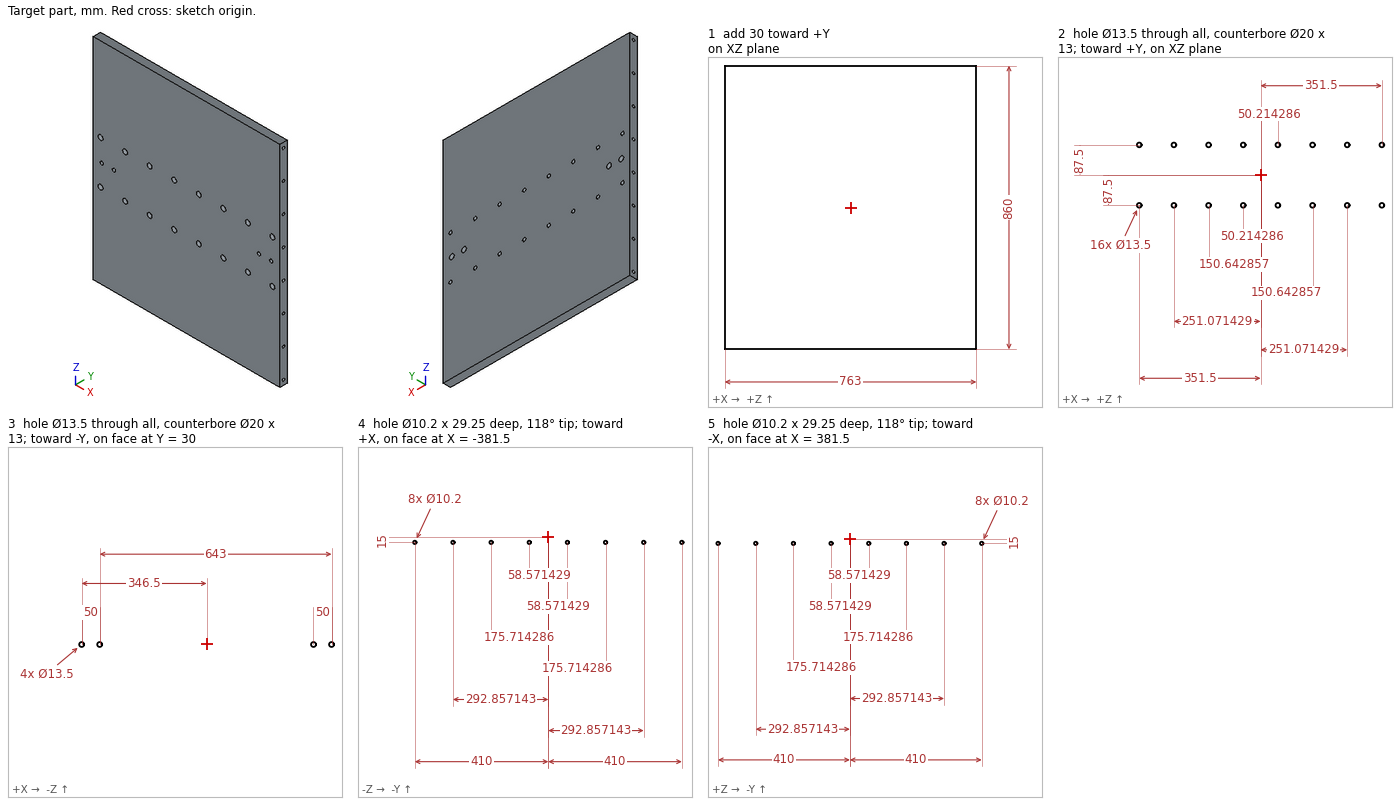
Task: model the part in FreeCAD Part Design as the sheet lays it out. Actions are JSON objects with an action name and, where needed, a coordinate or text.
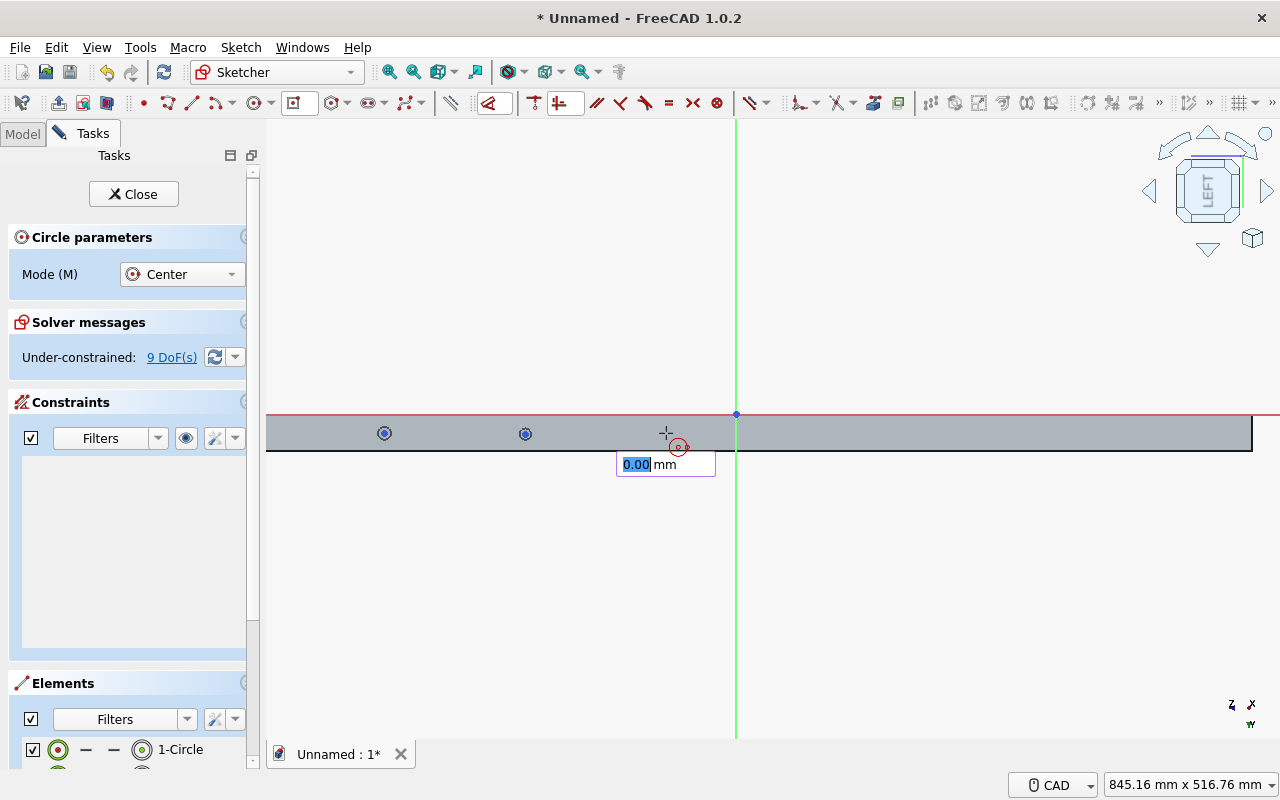
{"action": "scroll", "coordinate": [670, 437], "scroll_direction": "up", "scroll_amount": 5}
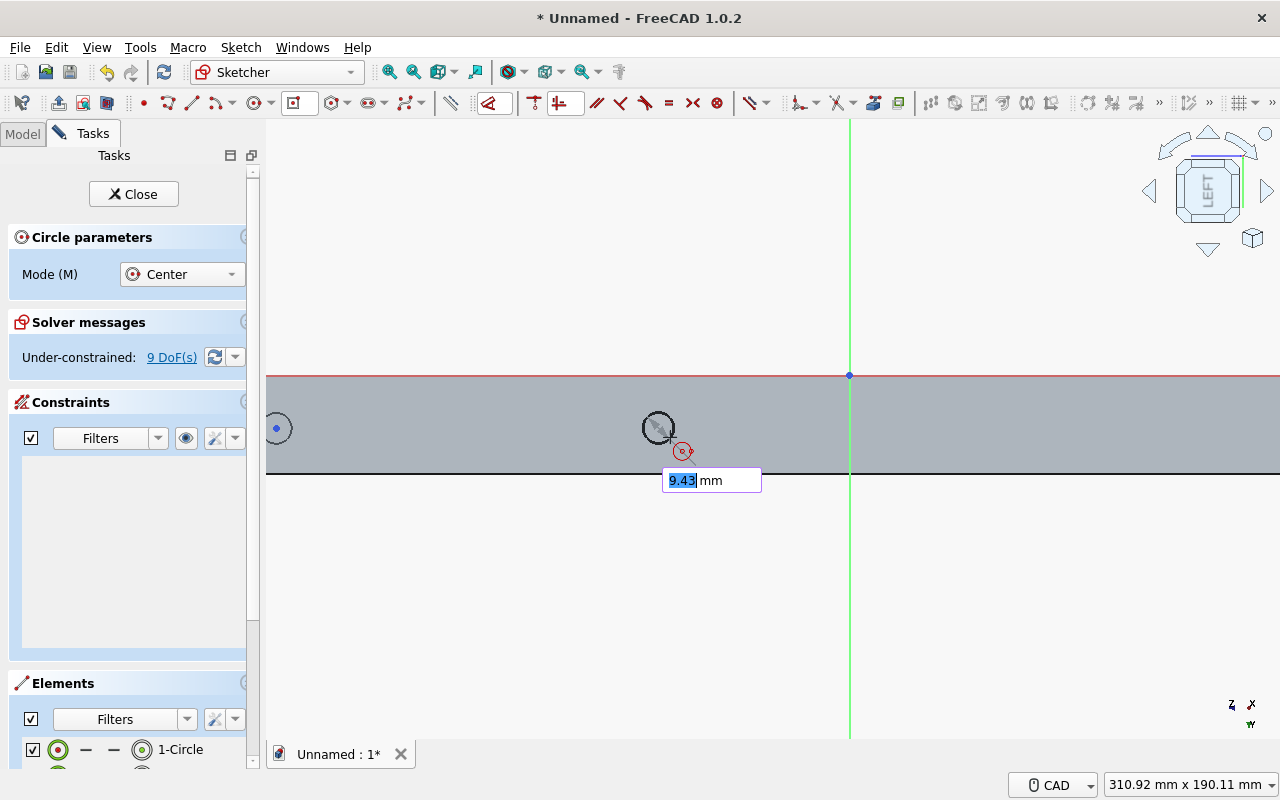
{"action": "left_click", "coordinate": [670, 436]}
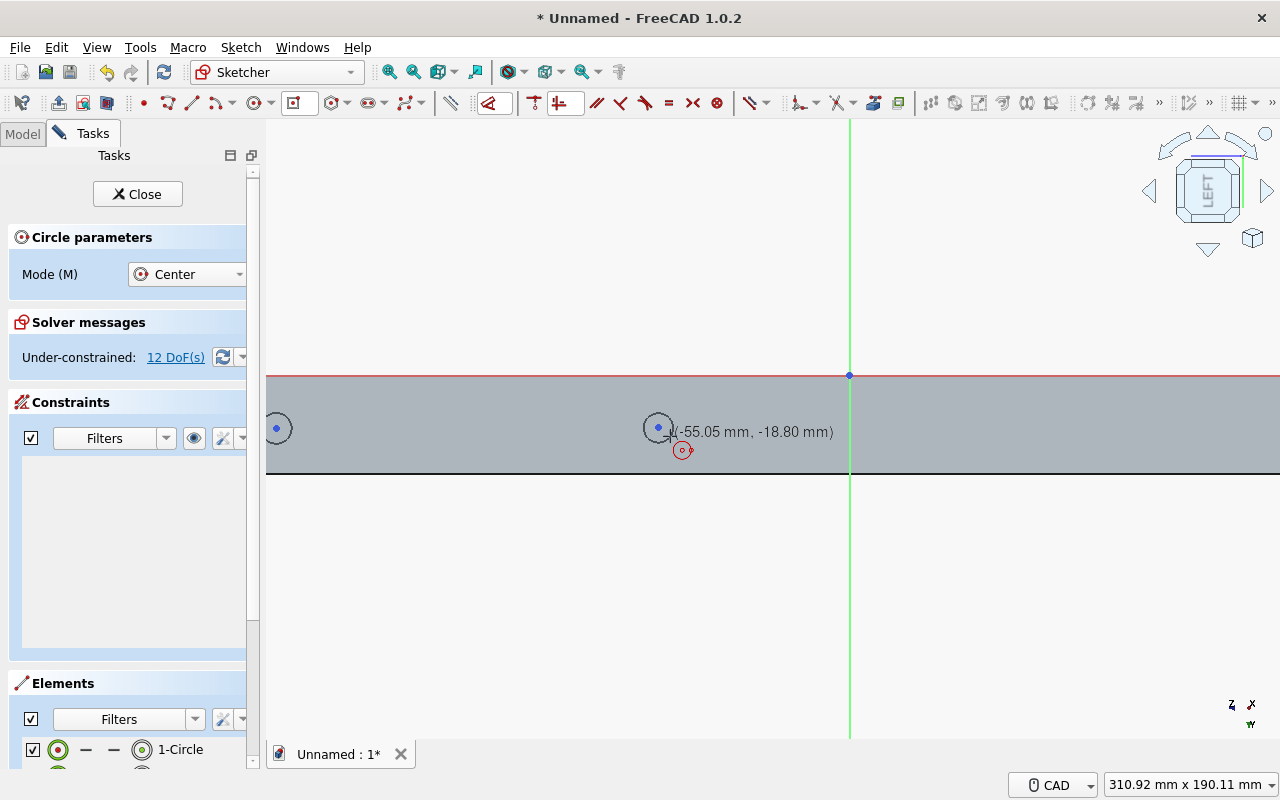
{"action": "scroll", "coordinate": [1041, 425], "scroll_direction": "up", "scroll_amount": 2}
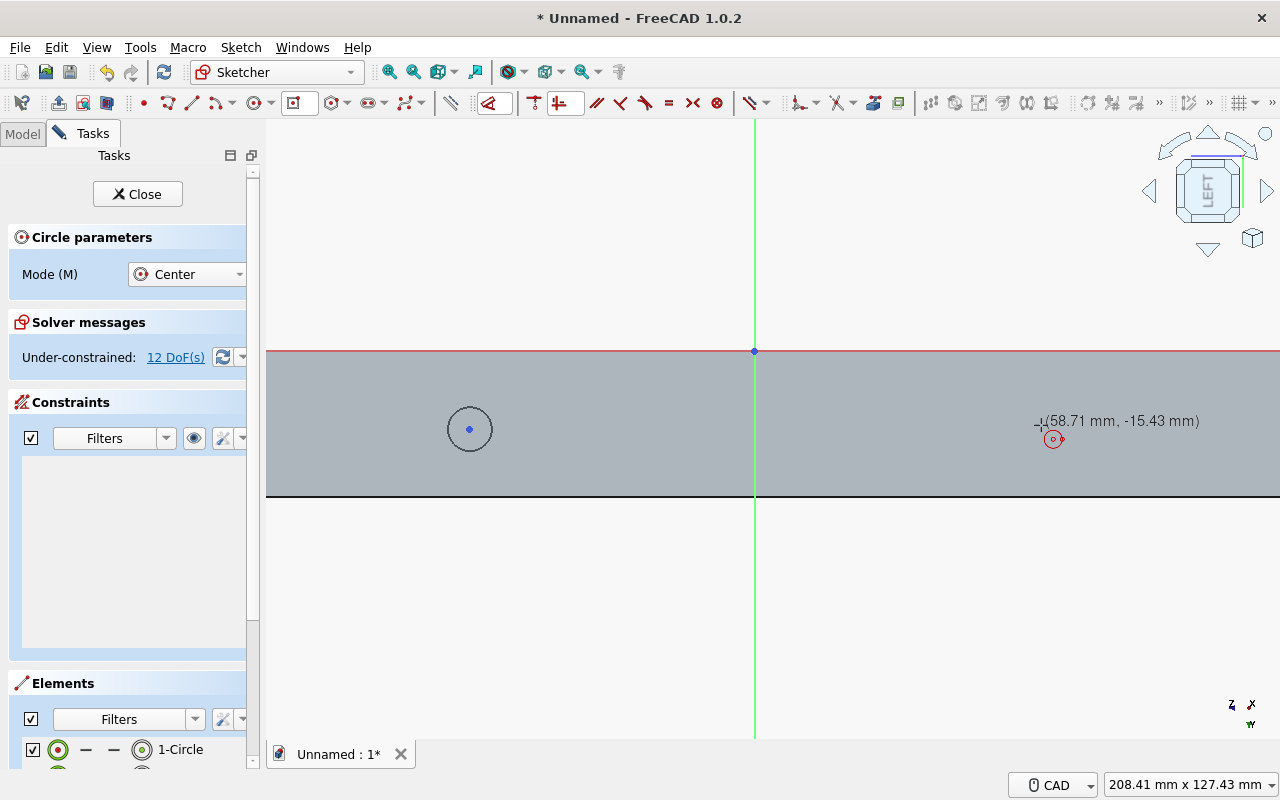
{"action": "scroll", "coordinate": [697, 434], "scroll_direction": "down", "scroll_amount": 10}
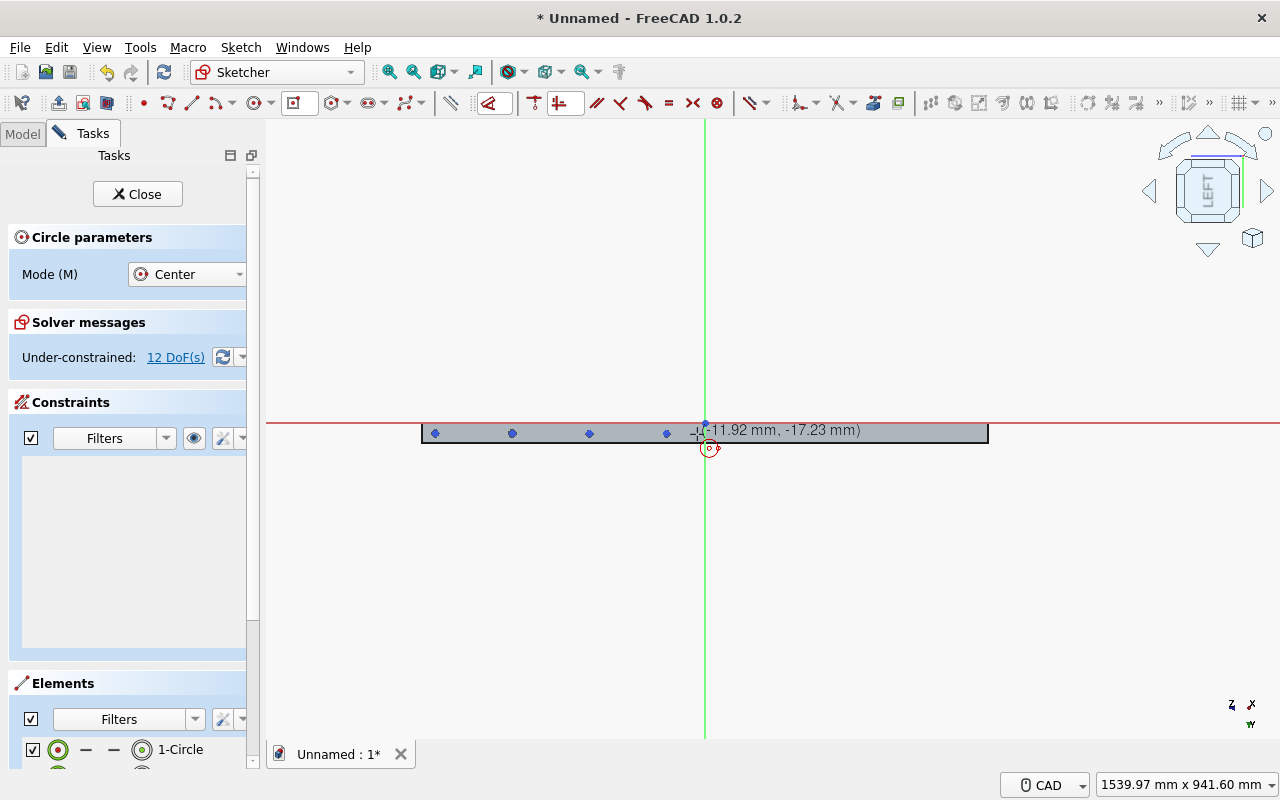
{"action": "scroll", "coordinate": [744, 433], "scroll_direction": "up", "scroll_amount": 3}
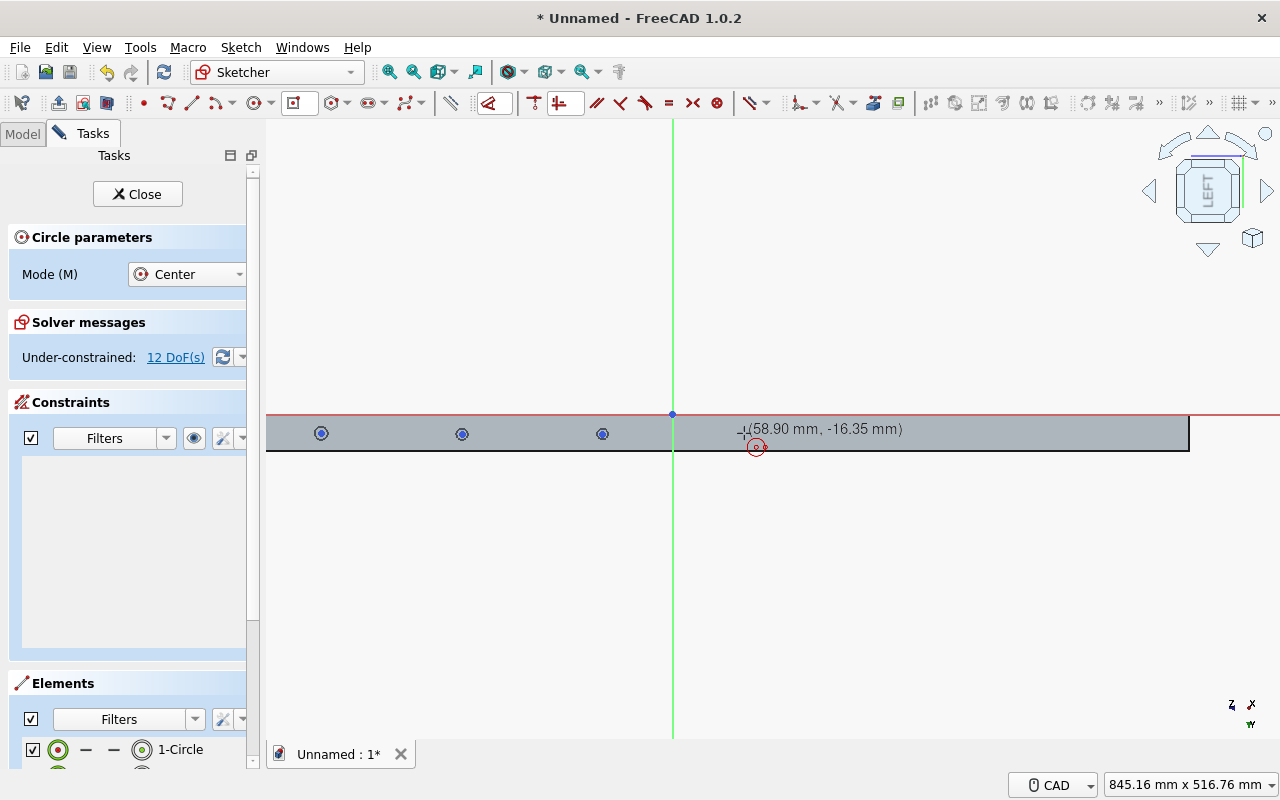
{"action": "left_click", "coordinate": [743, 433]}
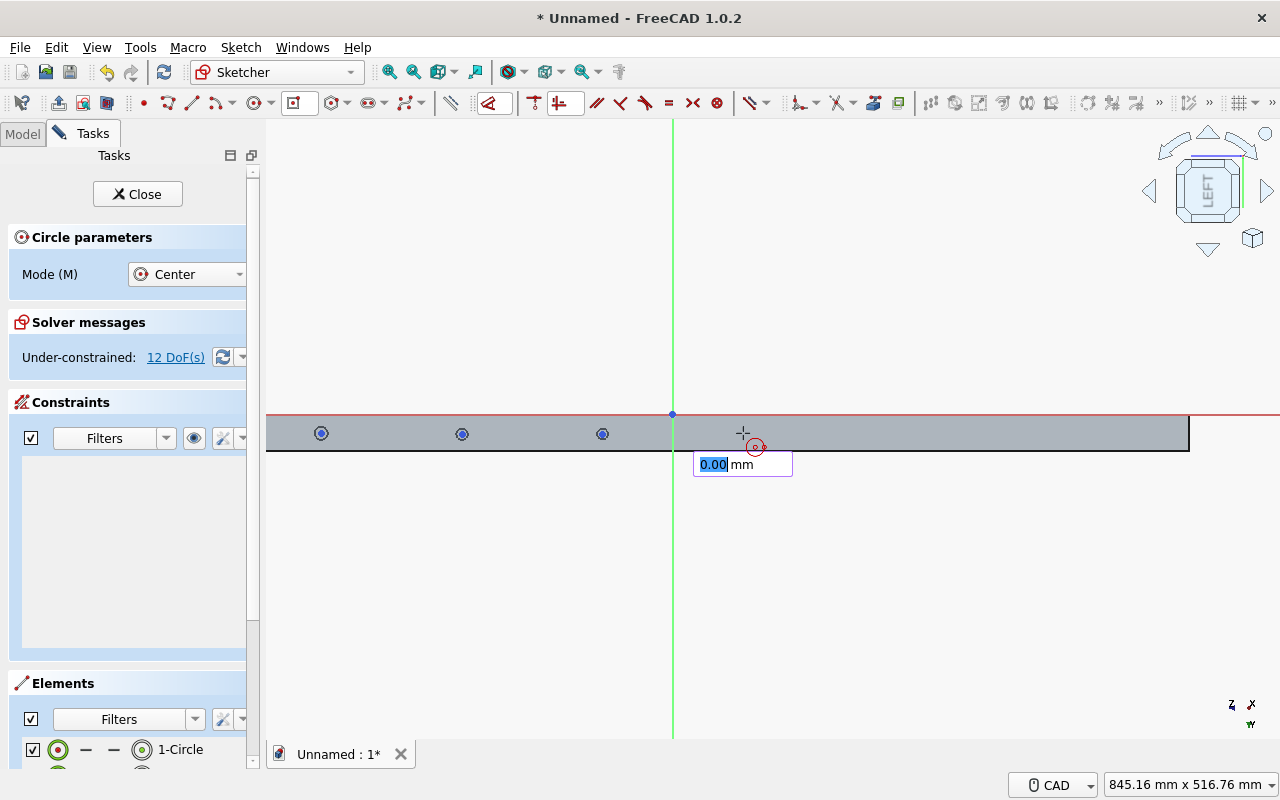
{"action": "scroll", "coordinate": [748, 437], "scroll_direction": "up", "scroll_amount": 5}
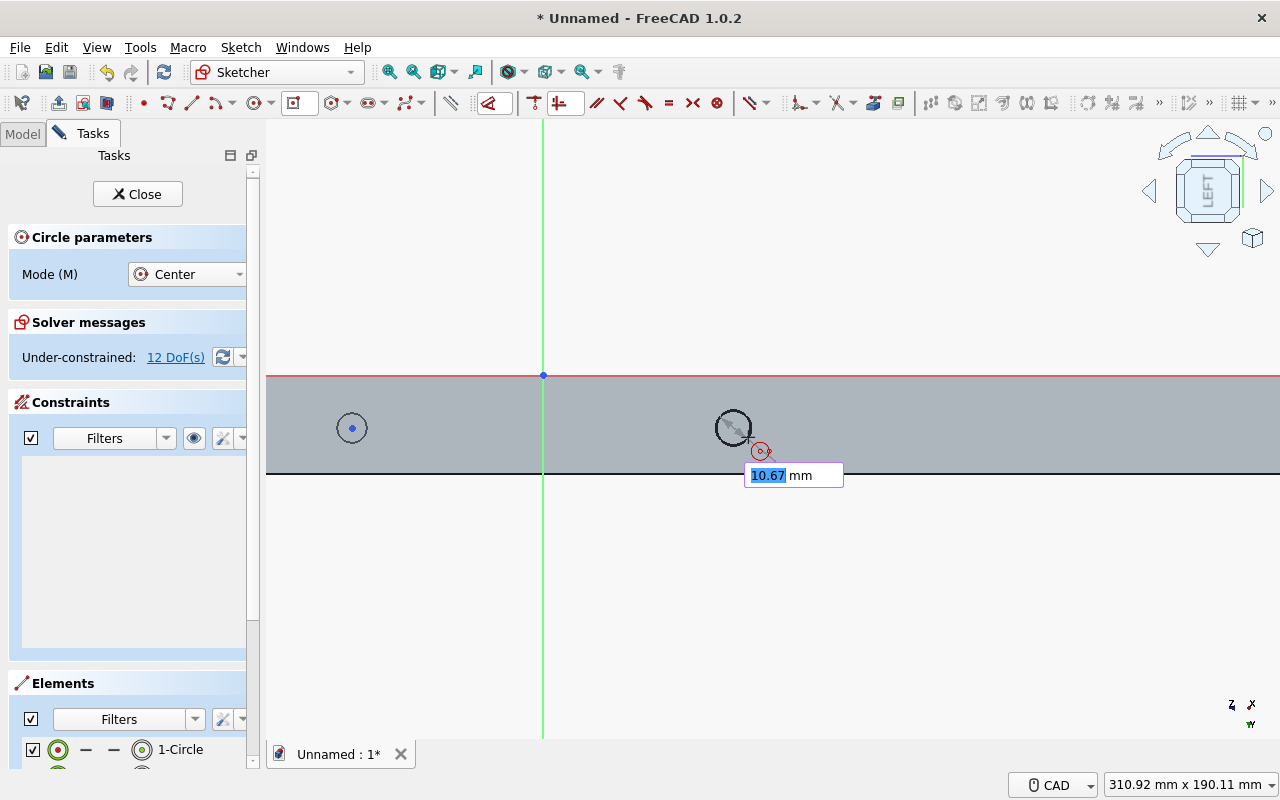
{"action": "left_click", "coordinate": [746, 436]}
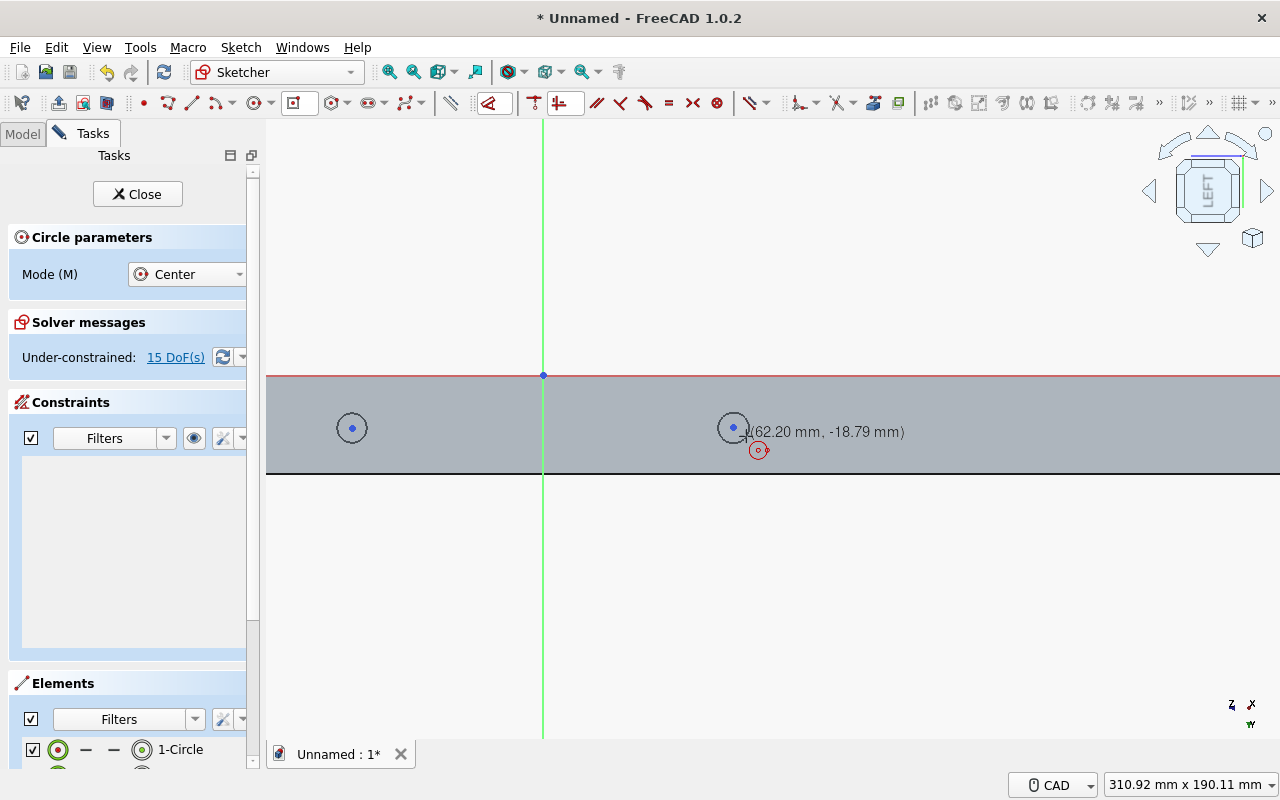
{"action": "scroll", "coordinate": [745, 434], "scroll_direction": "down", "scroll_amount": 8}